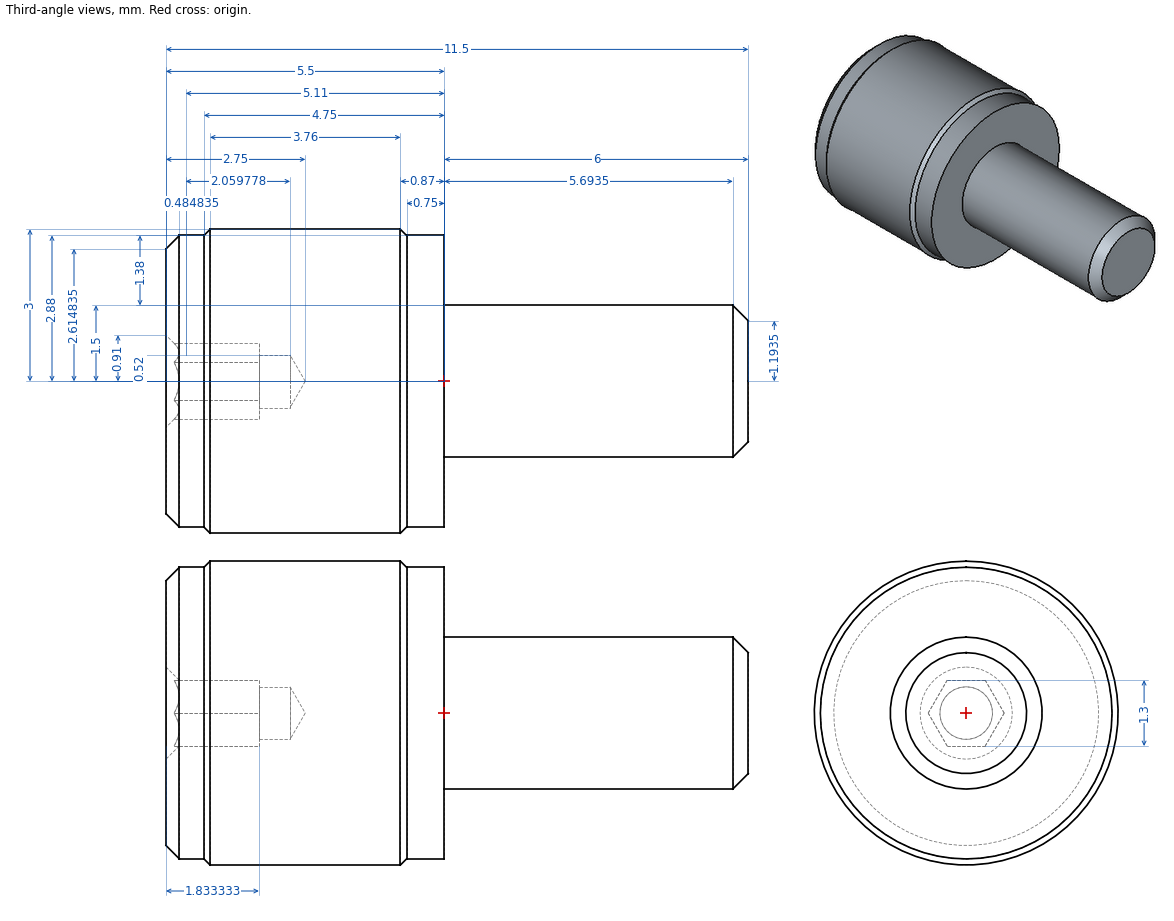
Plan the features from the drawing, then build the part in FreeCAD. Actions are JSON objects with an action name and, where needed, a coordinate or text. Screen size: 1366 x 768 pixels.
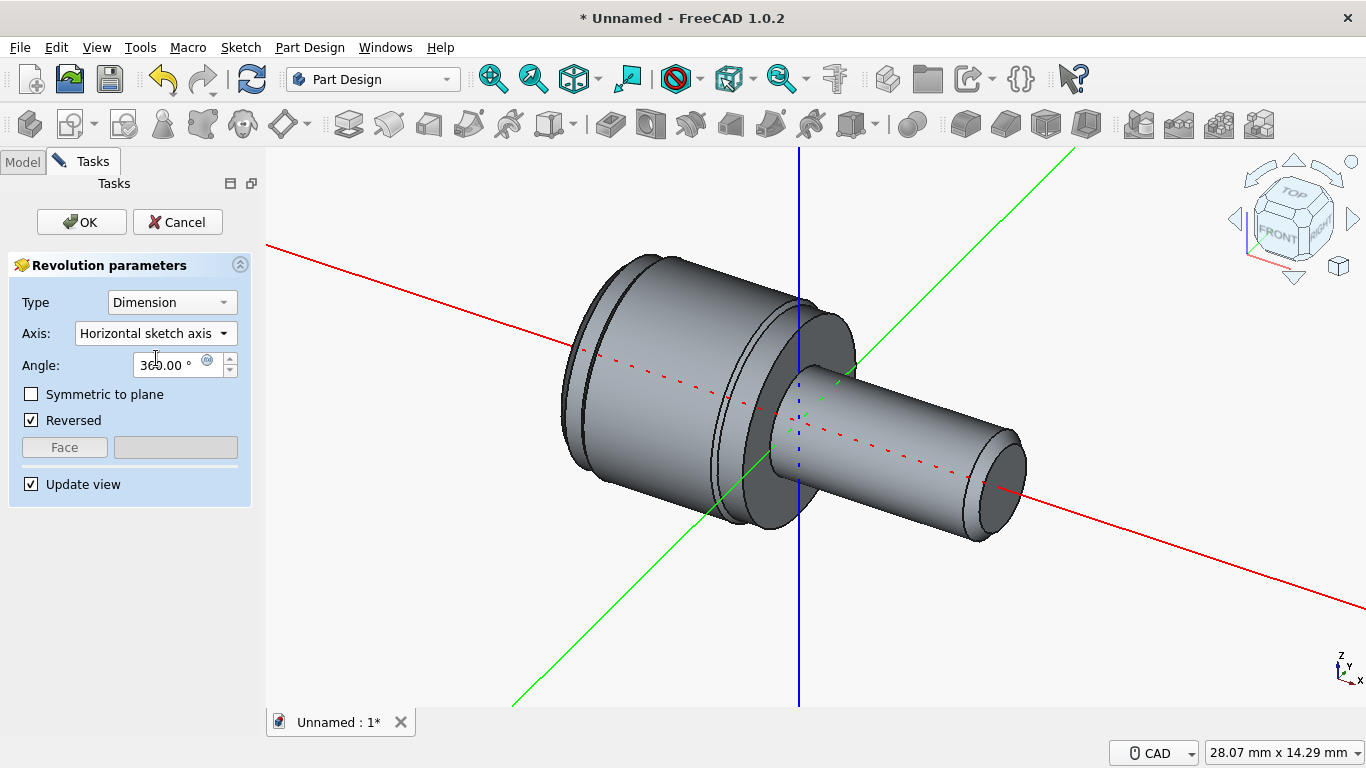
{"action": "left_click", "coordinate": [82, 222]}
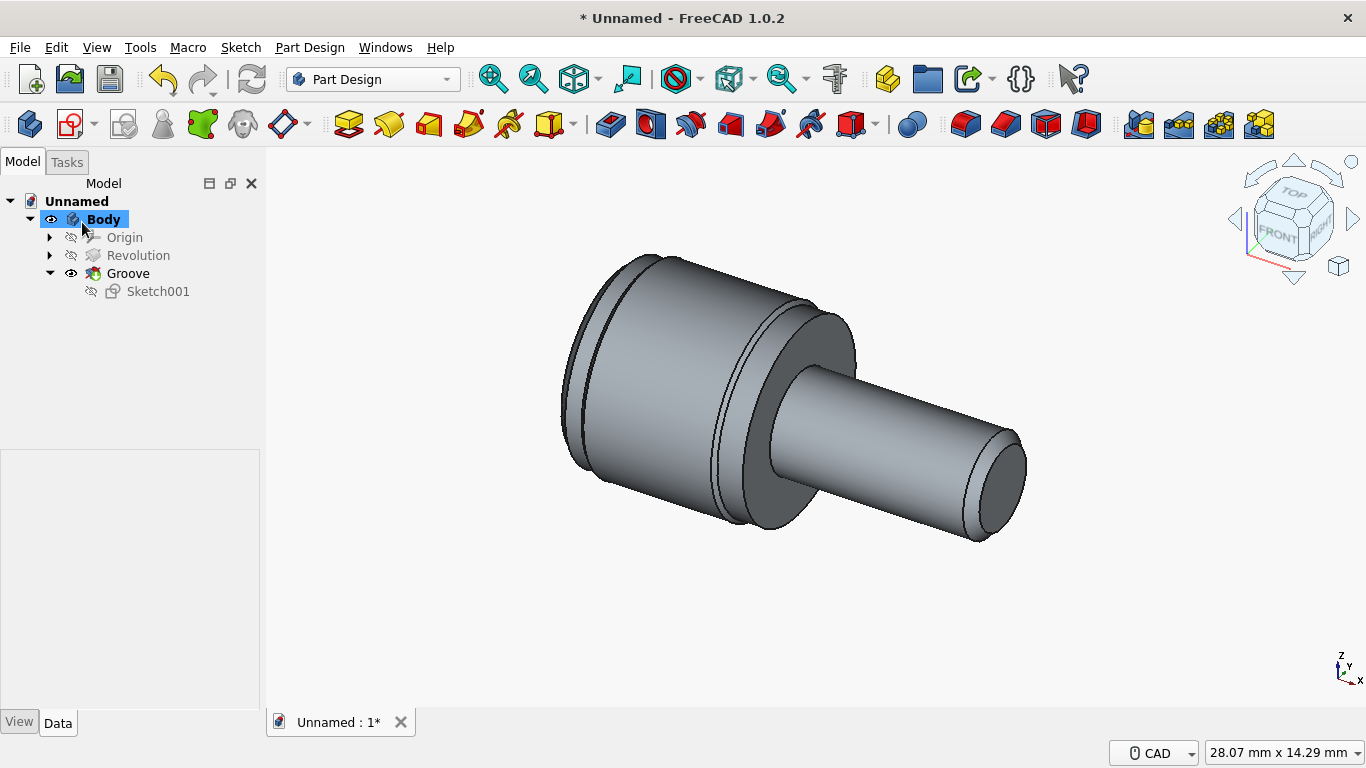
{"action": "key", "text": "6"}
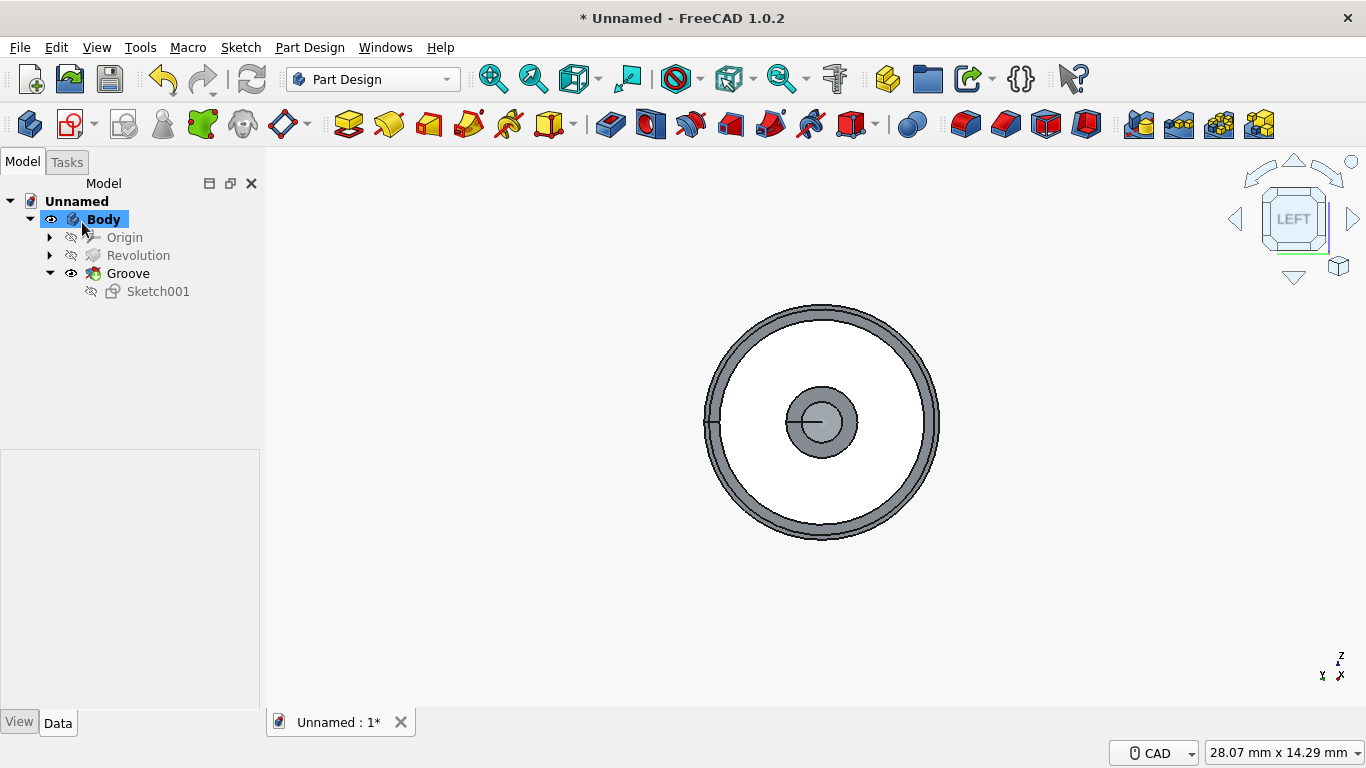
{"action": "left_click", "coordinate": [494, 80]}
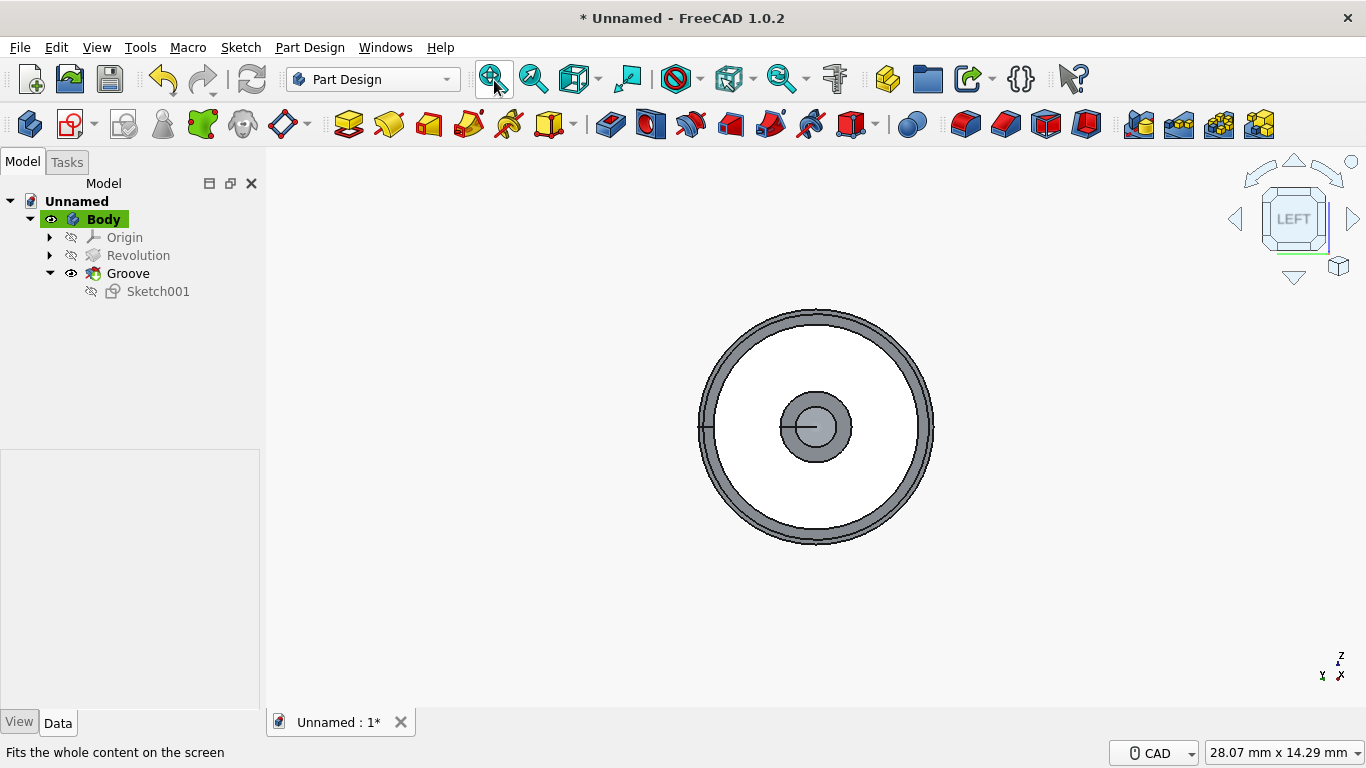
{"action": "left_click", "coordinate": [845, 367]}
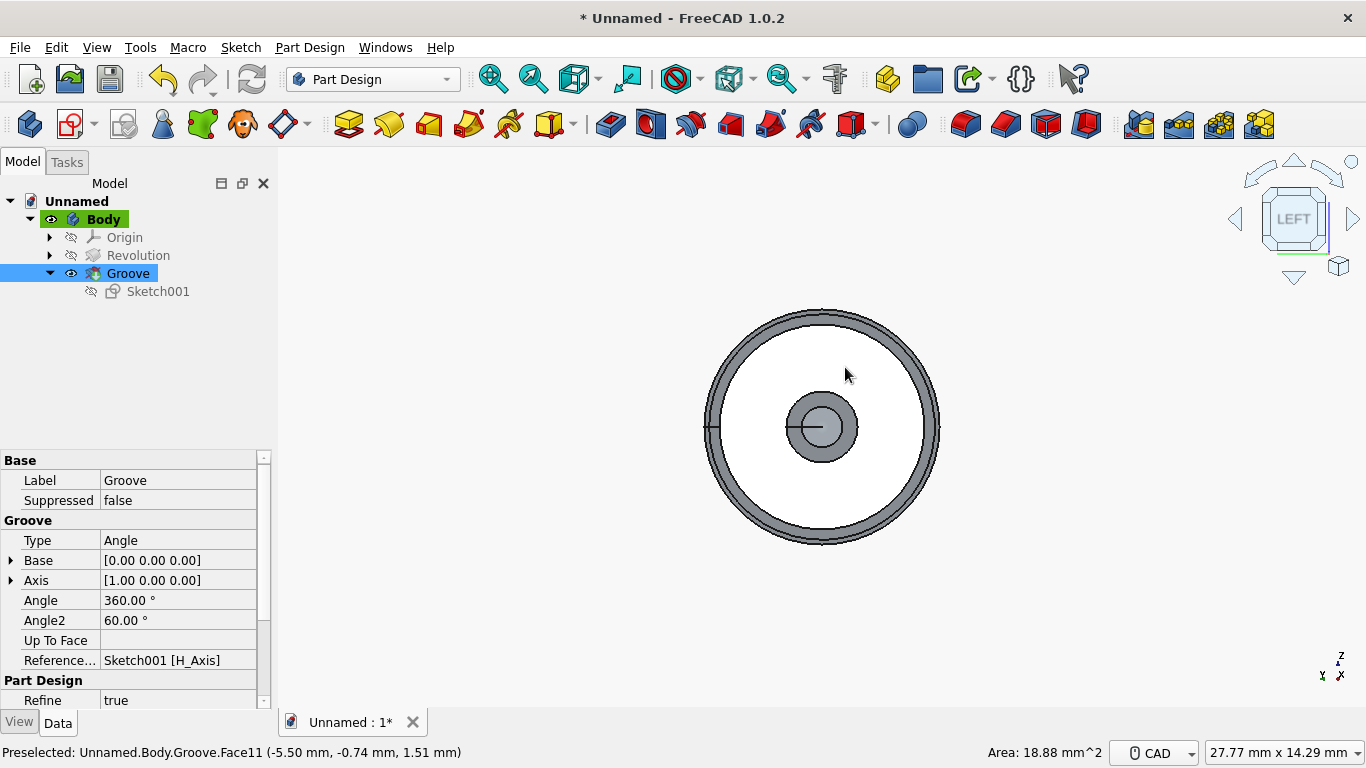
{"action": "left_click", "coordinate": [70, 124]}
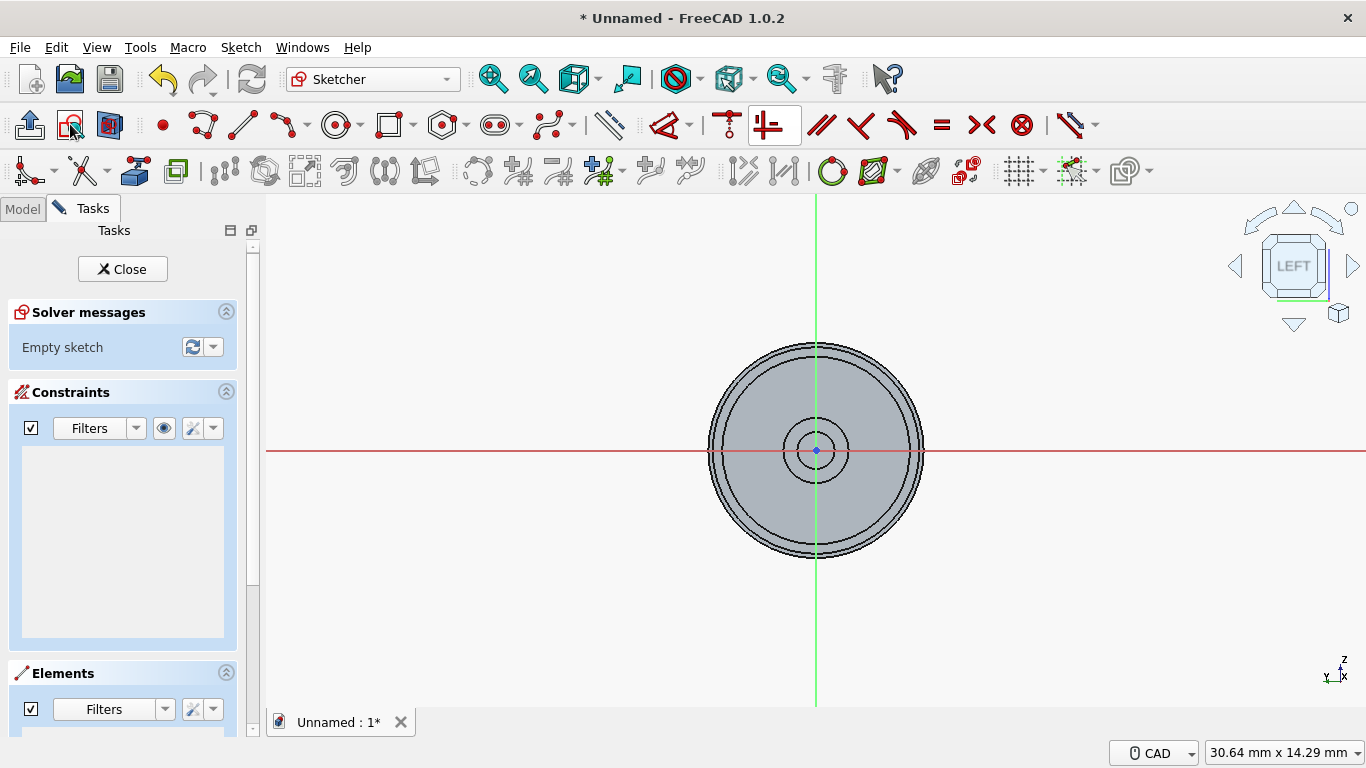
{"action": "scroll", "coordinate": [827, 450], "scroll_direction": "up", "scroll_amount": 10}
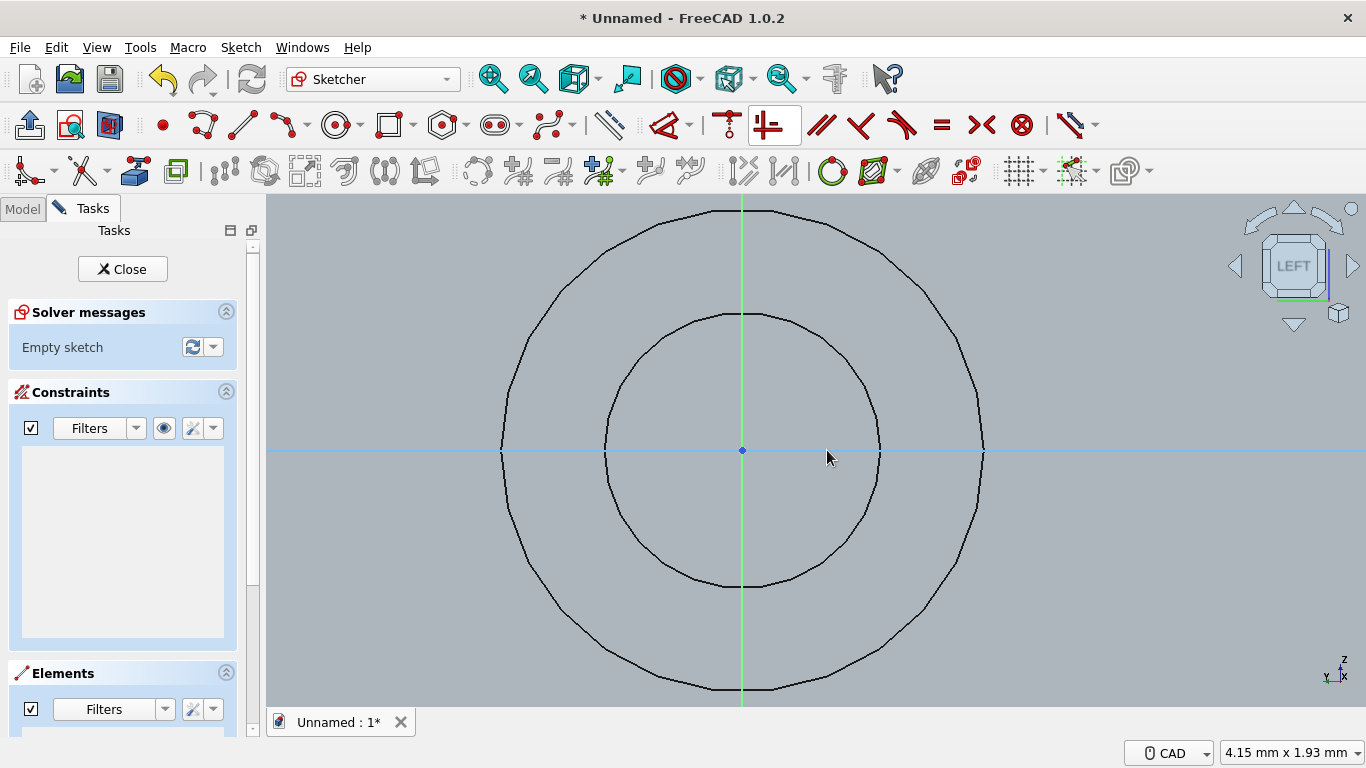
{"action": "left_click", "coordinate": [442, 126]}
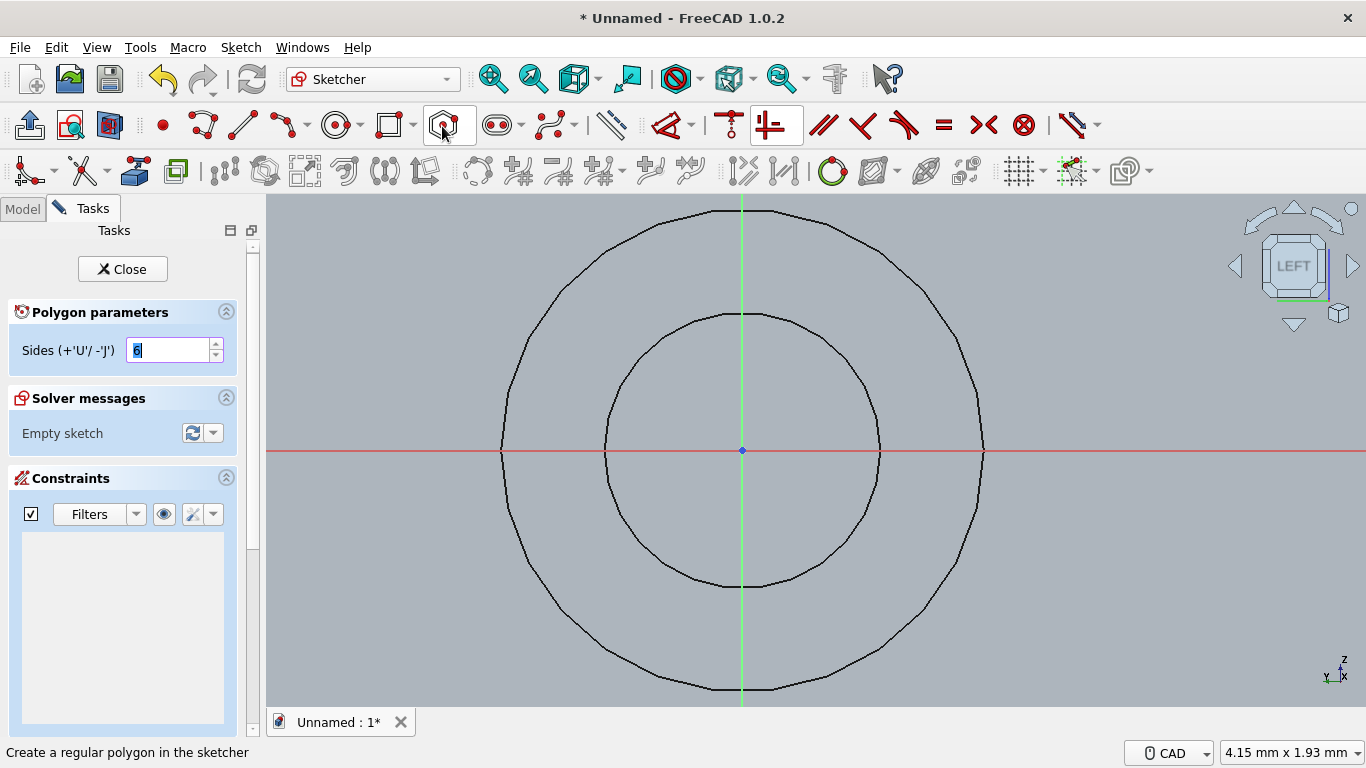
{"action": "left_click", "coordinate": [742, 450]}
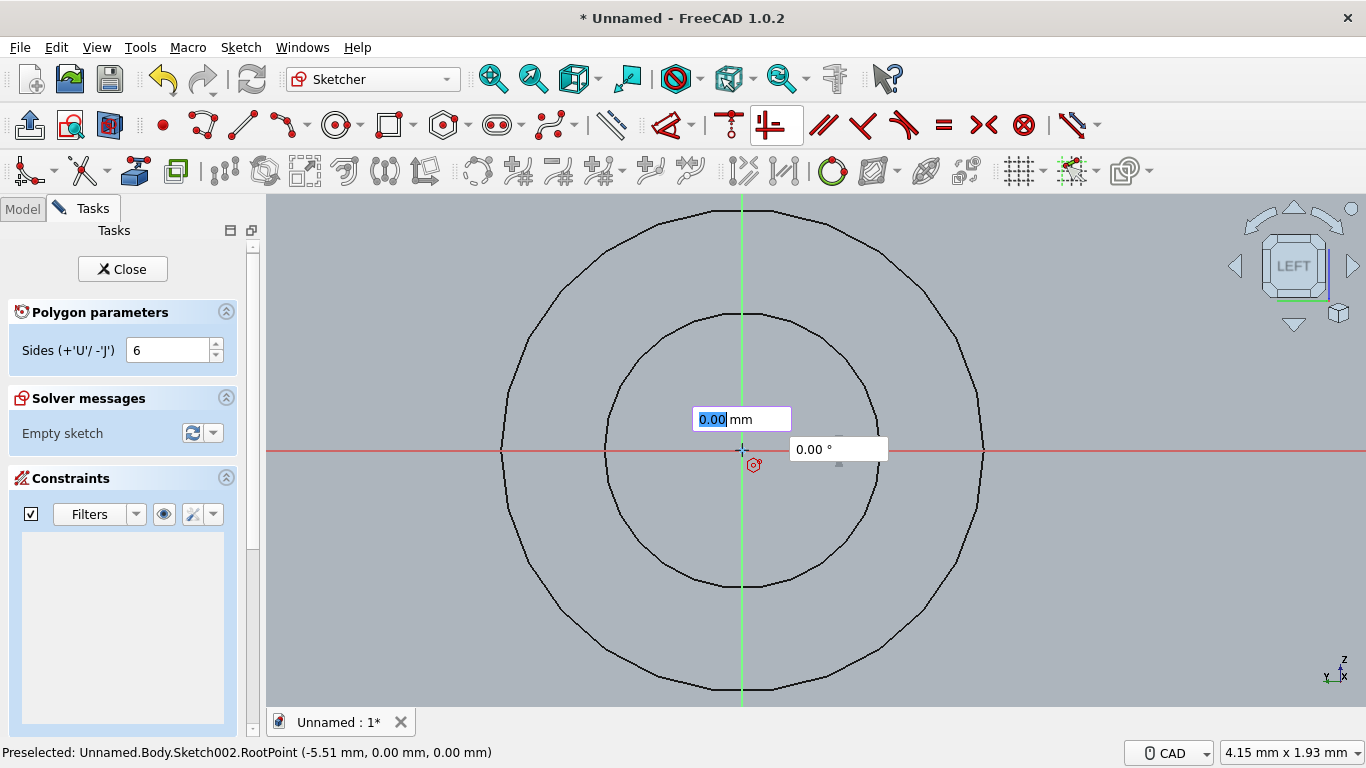
{"action": "left_click", "coordinate": [942, 450]}
{"action": "right_click", "coordinate": [942, 450]}